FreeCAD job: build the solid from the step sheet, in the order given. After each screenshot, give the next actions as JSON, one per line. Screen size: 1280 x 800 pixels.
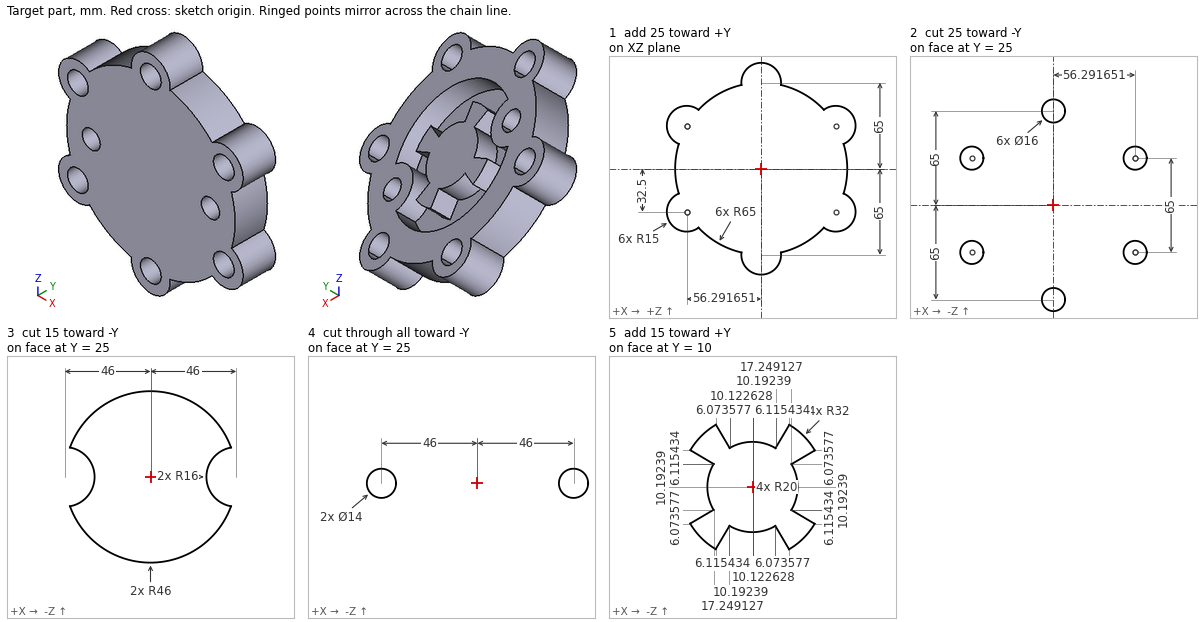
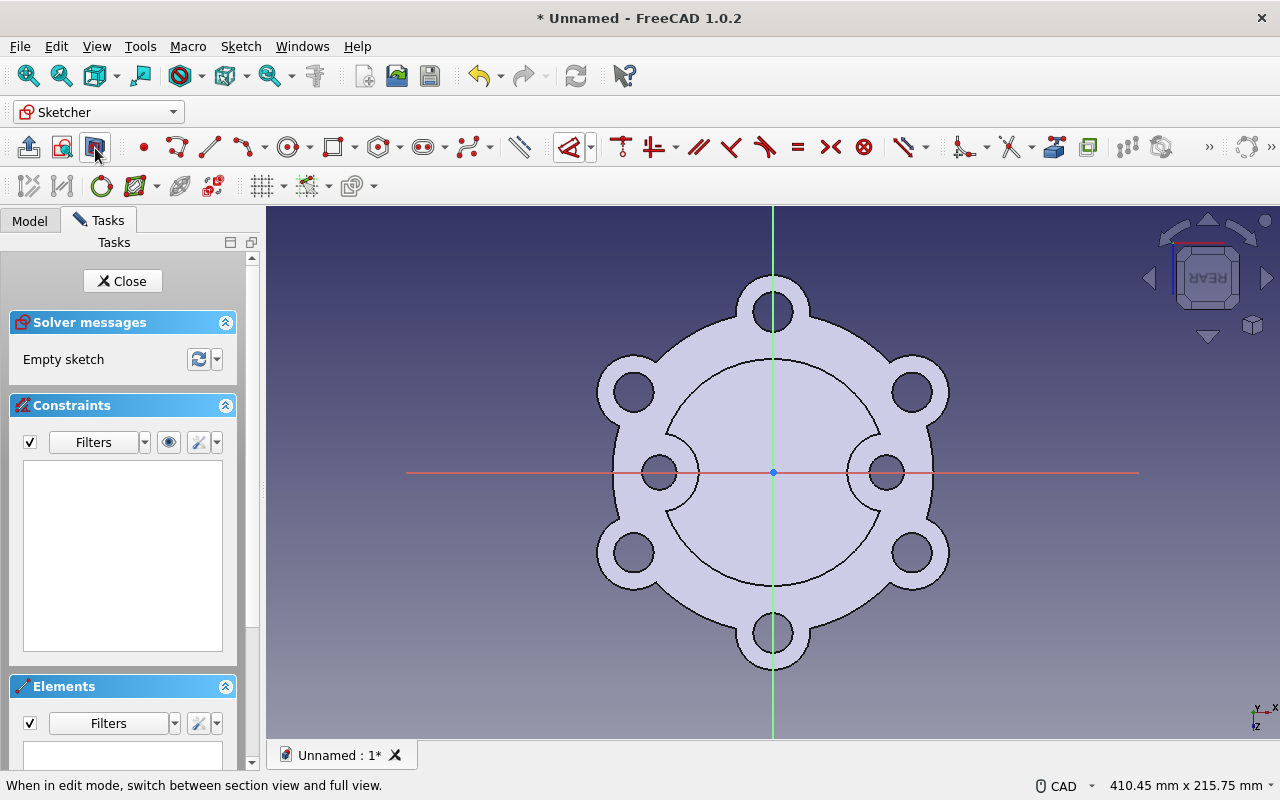
{"action": "scroll", "coordinate": [813, 472], "scroll_direction": "up", "scroll_amount": 5}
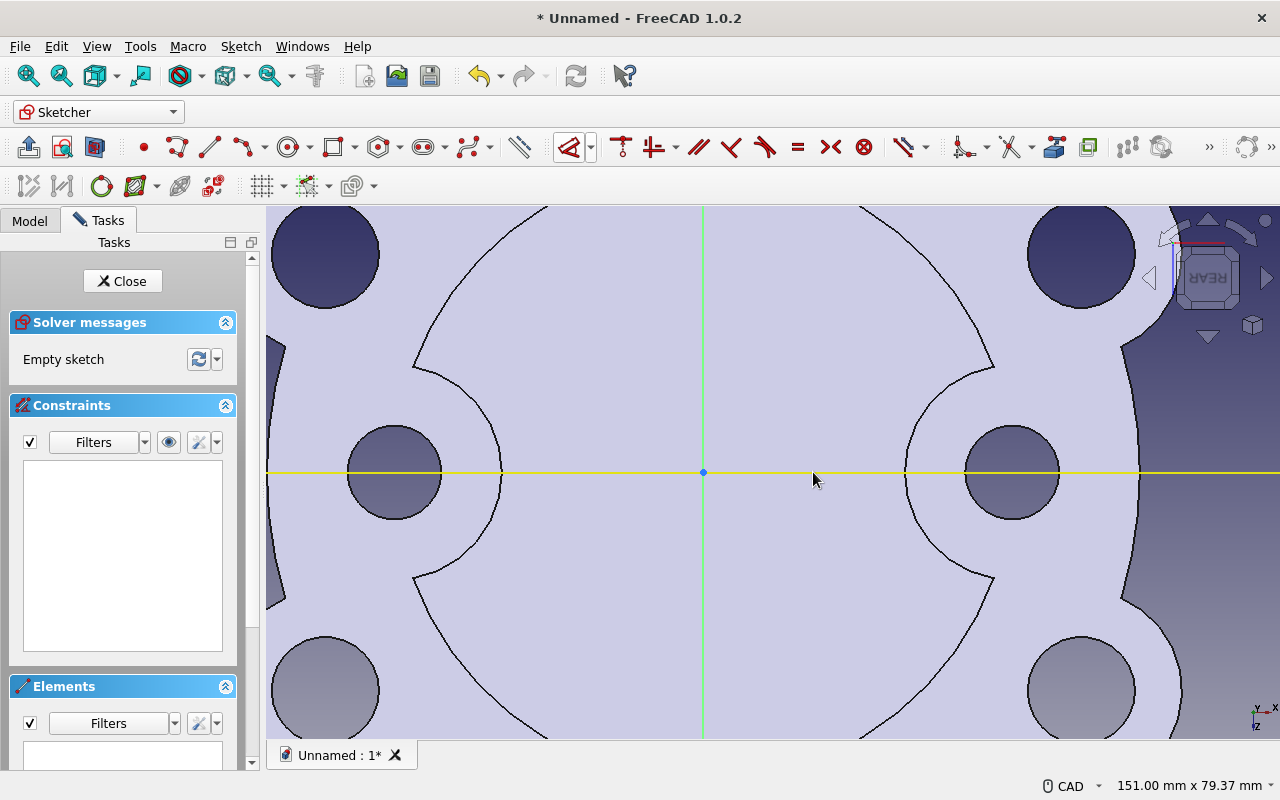
{"action": "left_click", "coordinate": [210, 148]}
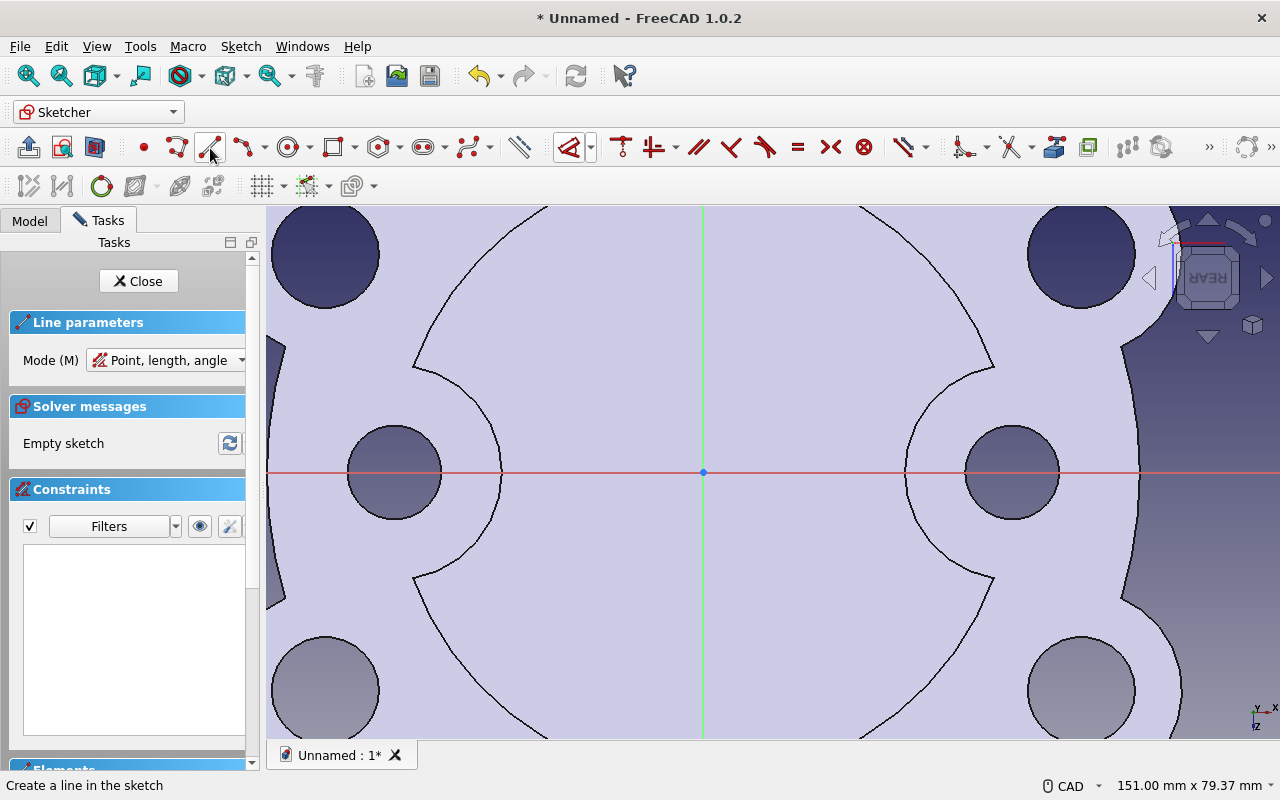
{"action": "left_click", "coordinate": [888, 582]}
{"action": "left_click", "coordinate": [819, 541]}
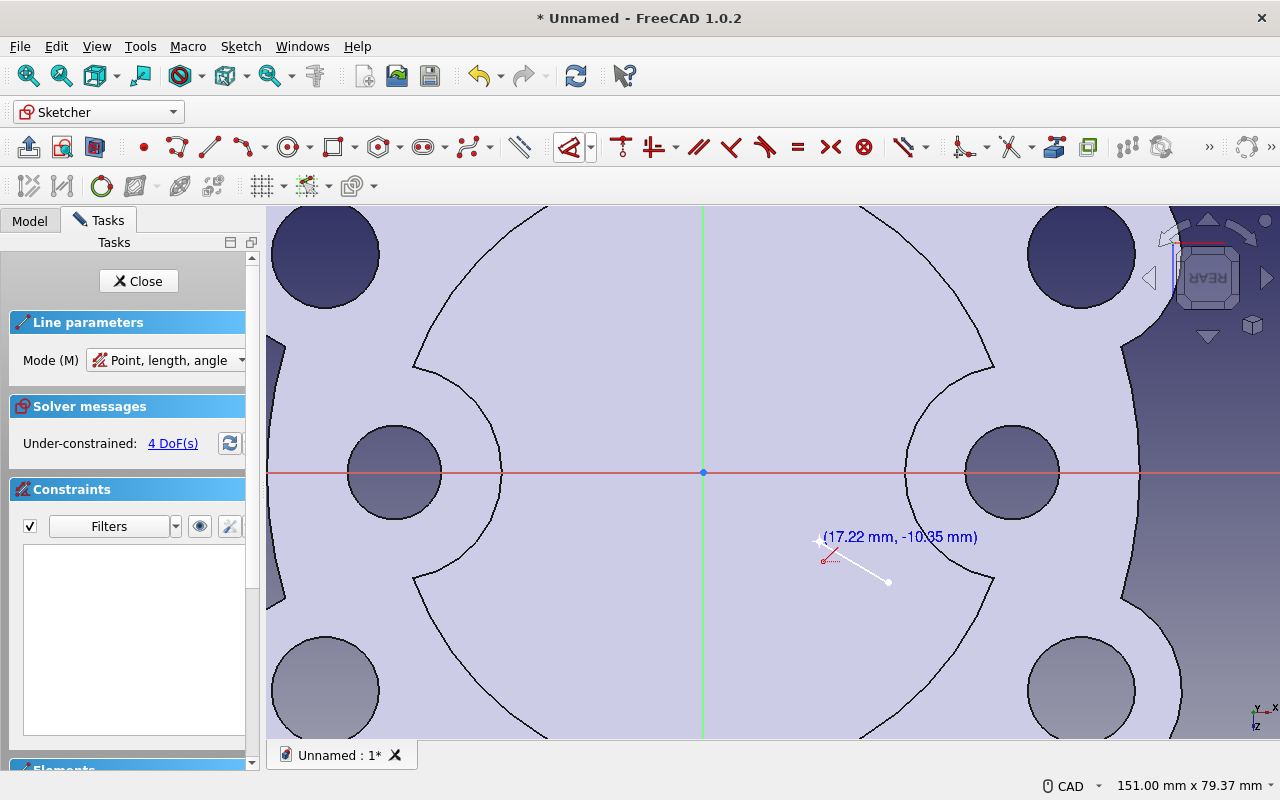
{"action": "left_click", "coordinate": [819, 405]}
{"action": "left_click", "coordinate": [889, 364]}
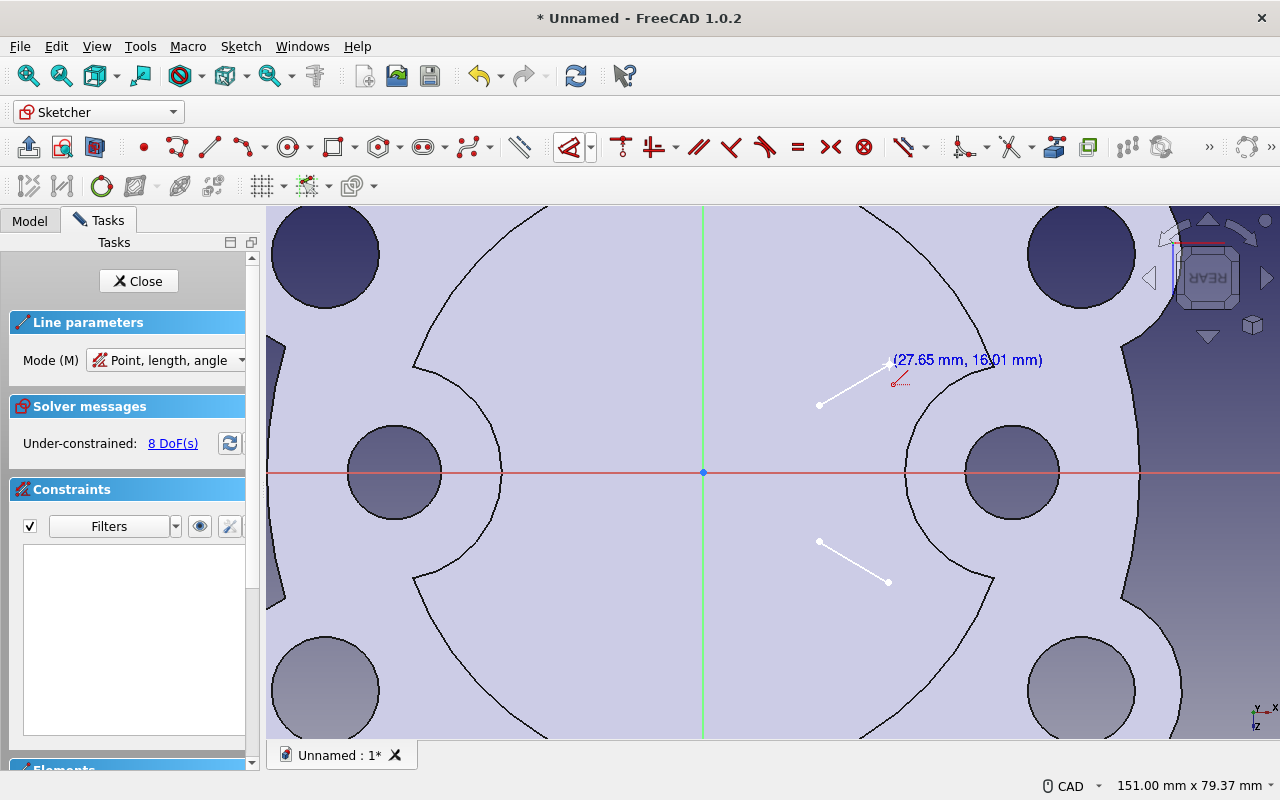
{"action": "left_click", "coordinate": [813, 288]}
{"action": "left_click", "coordinate": [772, 357]}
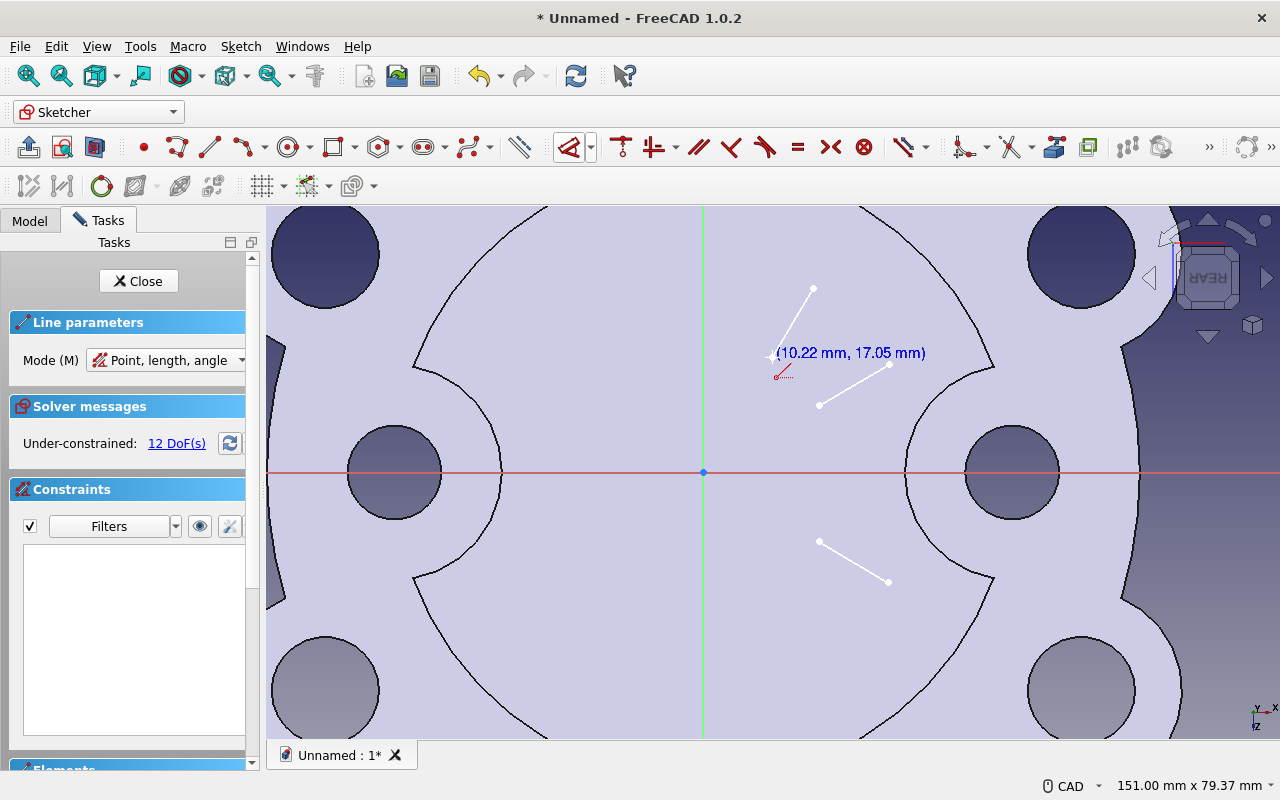
{"action": "left_click", "coordinate": [635, 357]}
{"action": "left_click", "coordinate": [595, 287]}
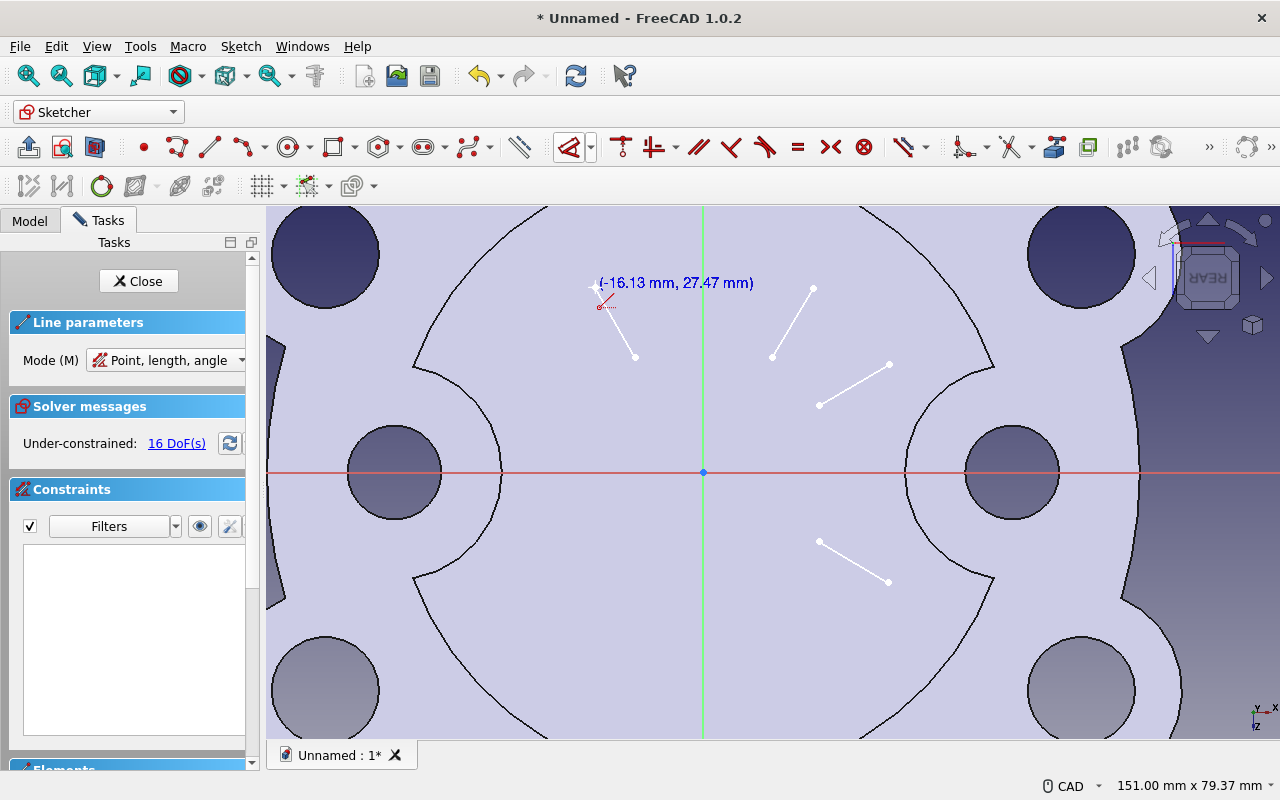
{"action": "left_click", "coordinate": [518, 363]}
{"action": "left_click", "coordinate": [588, 404]}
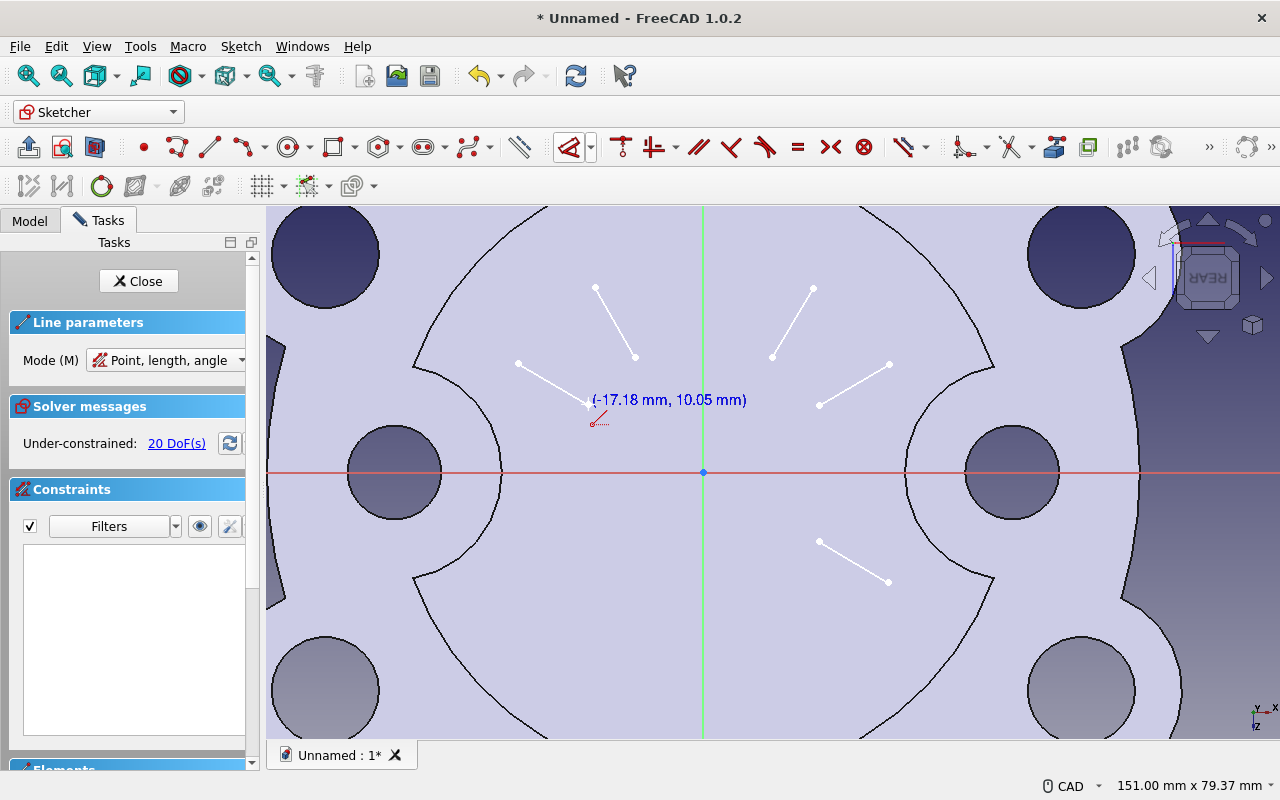
{"action": "left_click", "coordinate": [588, 540]}
{"action": "left_click", "coordinate": [518, 581]}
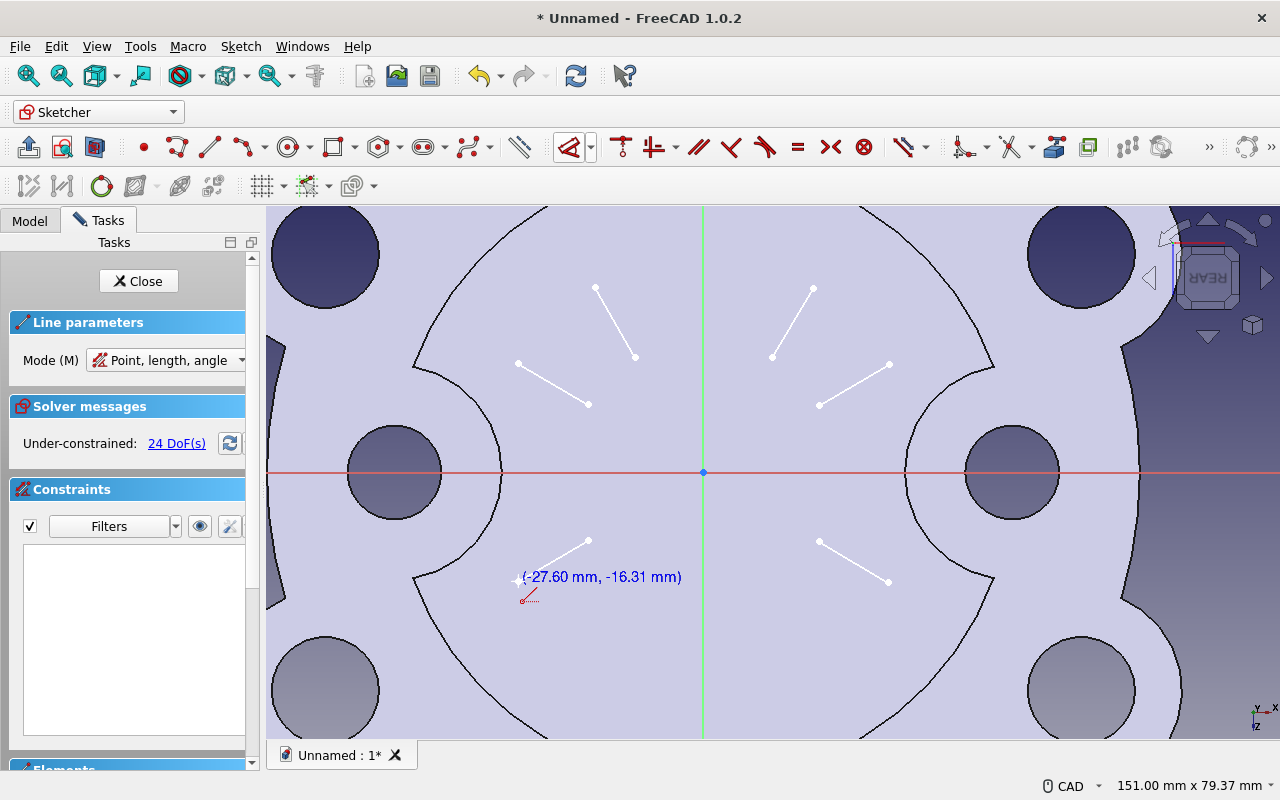
{"action": "left_click", "coordinate": [594, 657]}
{"action": "left_click", "coordinate": [635, 588]}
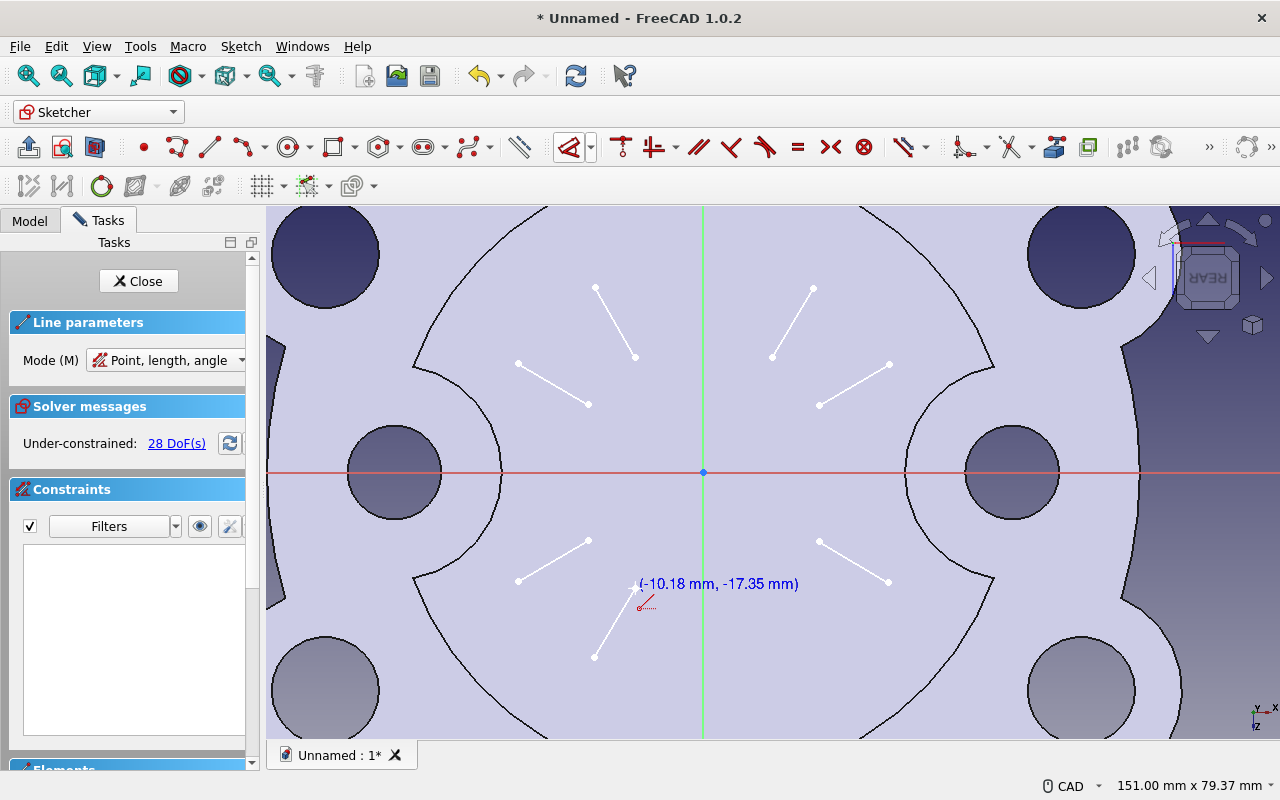
{"action": "left_click", "coordinate": [771, 588]}
{"action": "left_click", "coordinate": [812, 658]}